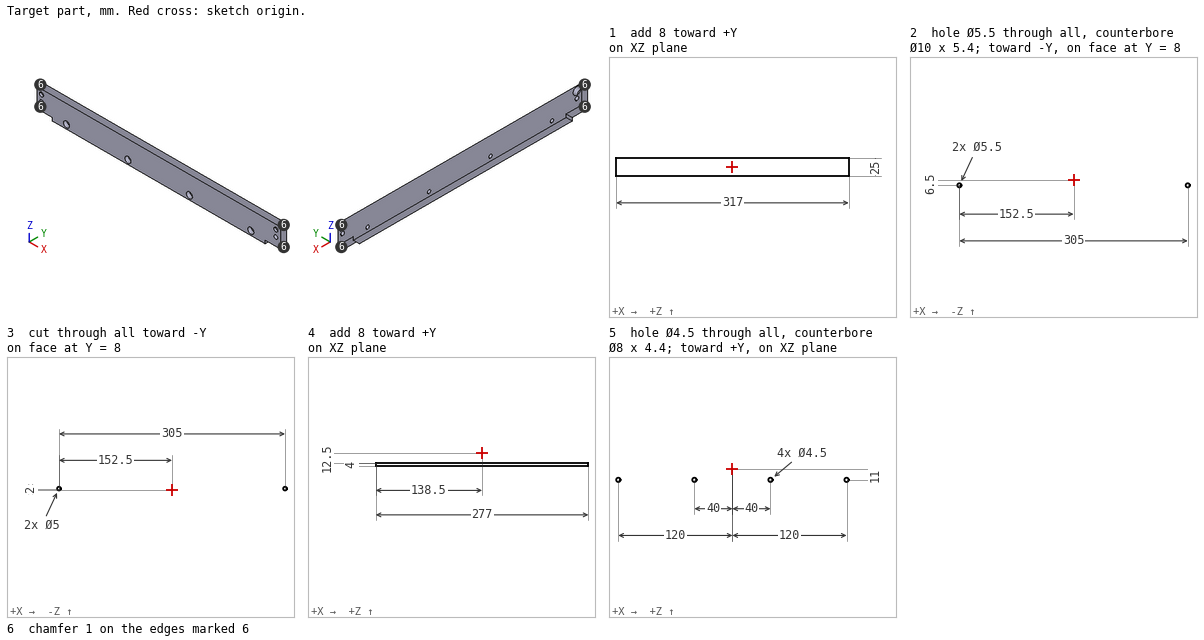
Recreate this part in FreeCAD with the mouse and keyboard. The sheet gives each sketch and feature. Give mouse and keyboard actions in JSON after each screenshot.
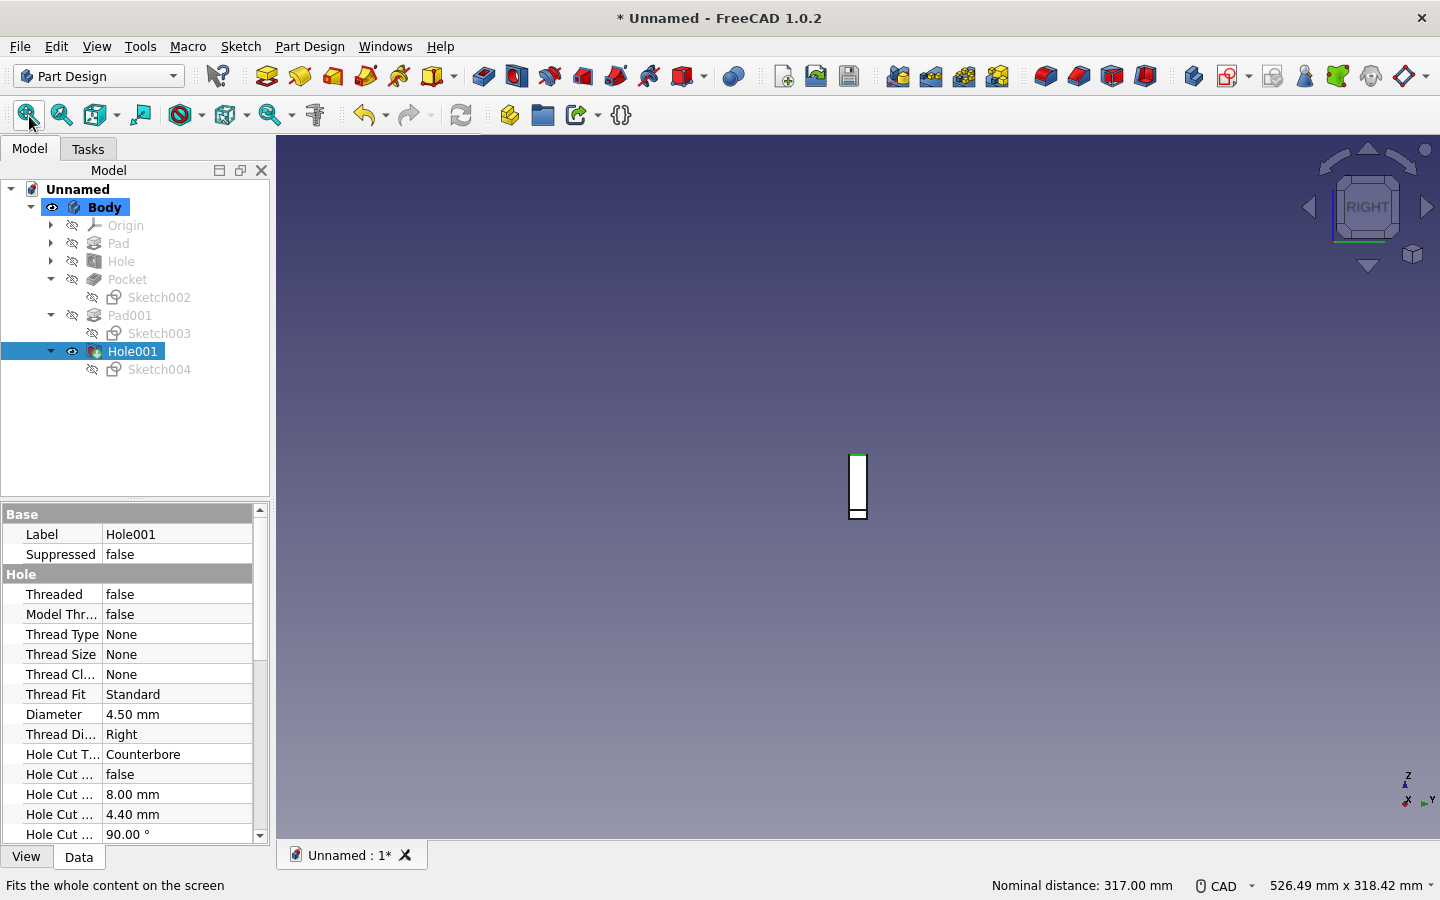
{"action": "left_click", "coordinate": [858, 509], "text": "ctrl"}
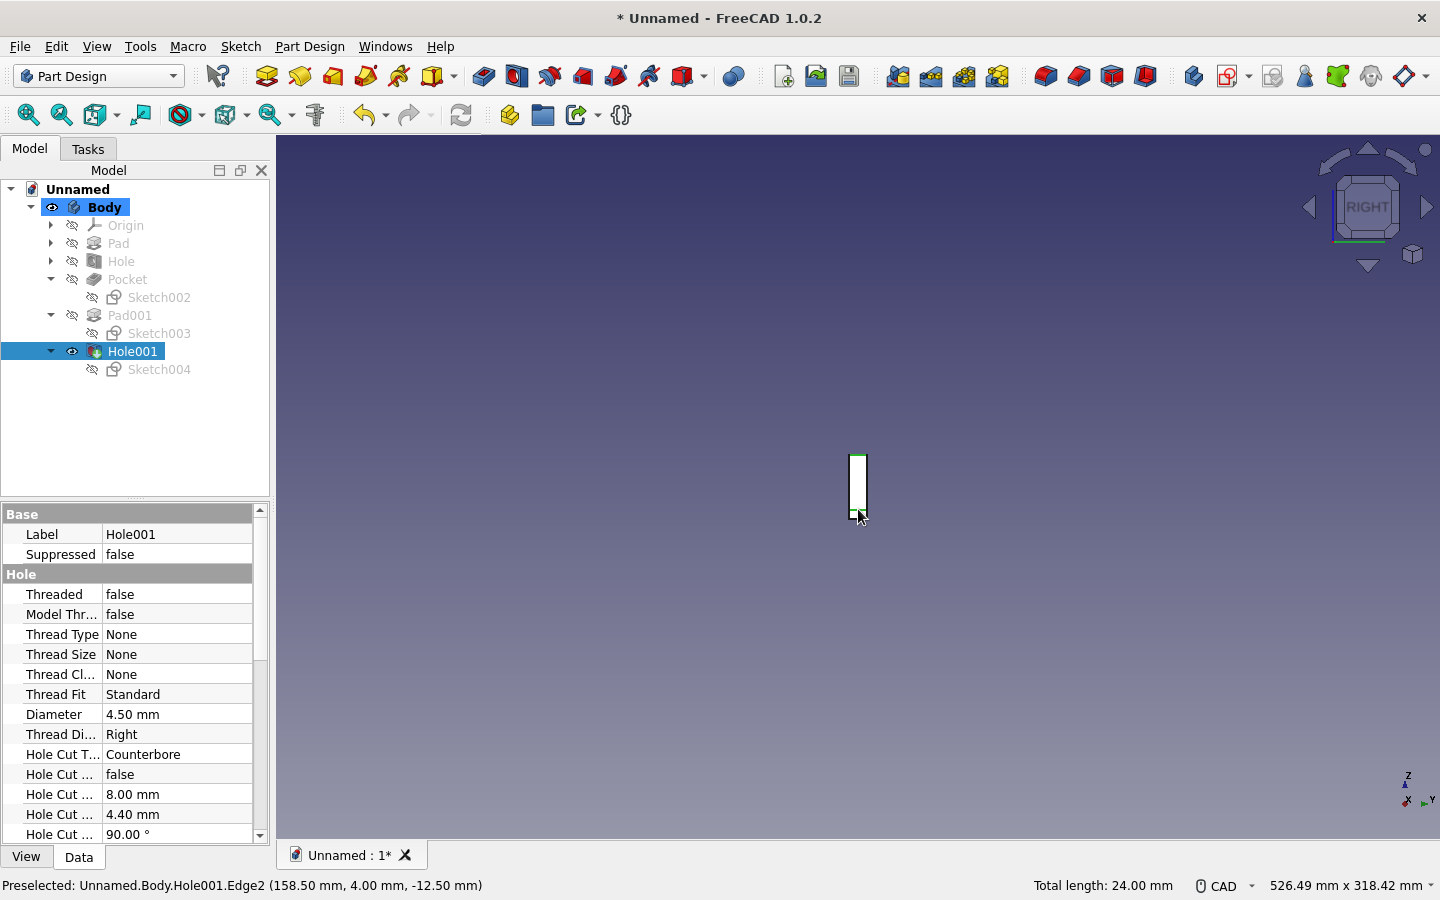
{"action": "scroll", "coordinate": [858, 509], "scroll_direction": "up", "scroll_amount": 5}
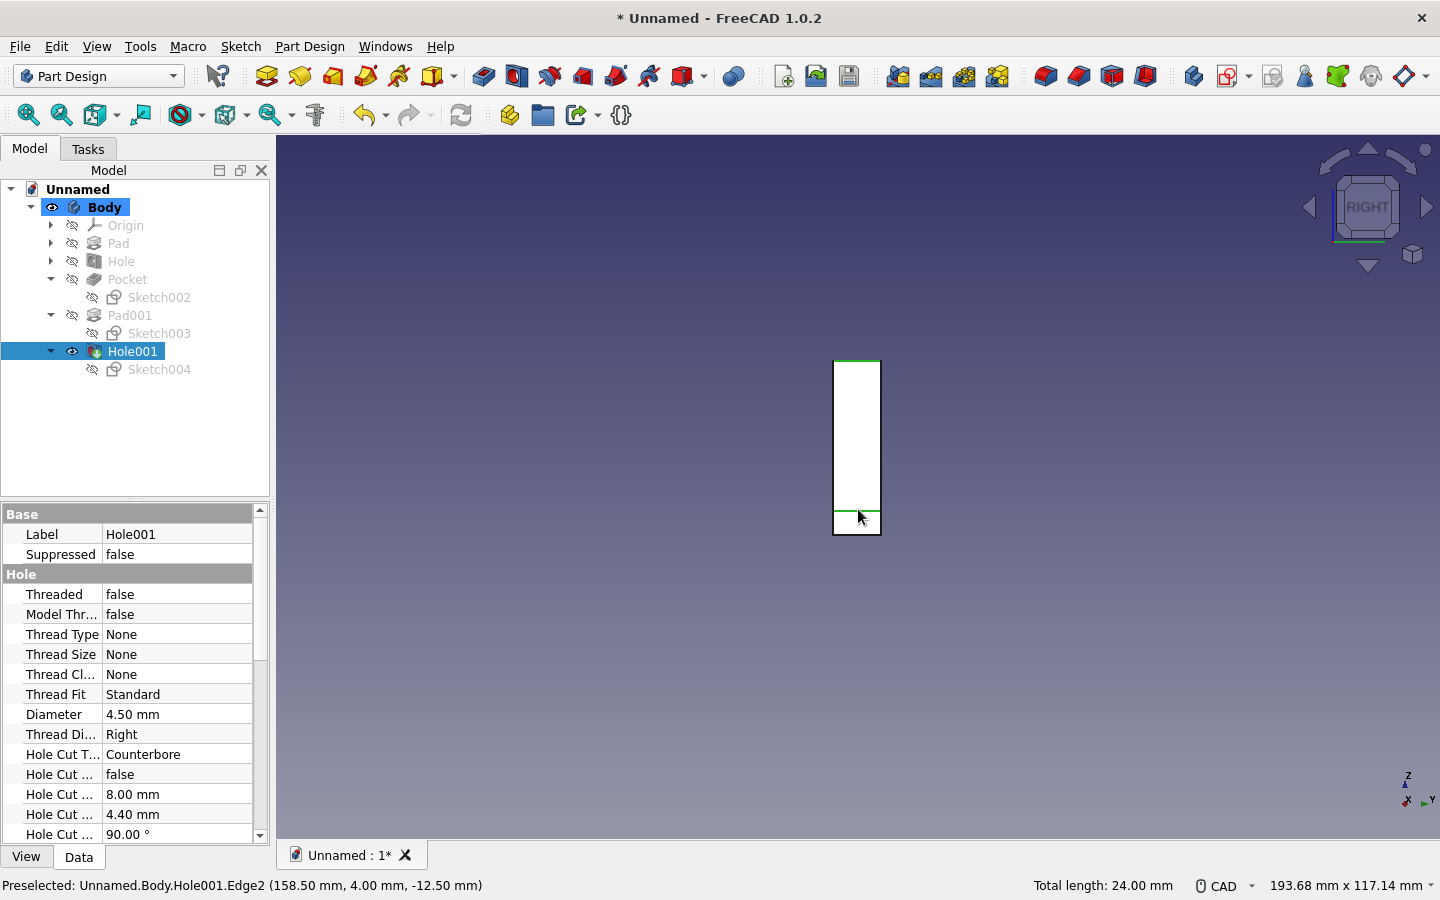
{"action": "left_click", "coordinate": [29, 116]}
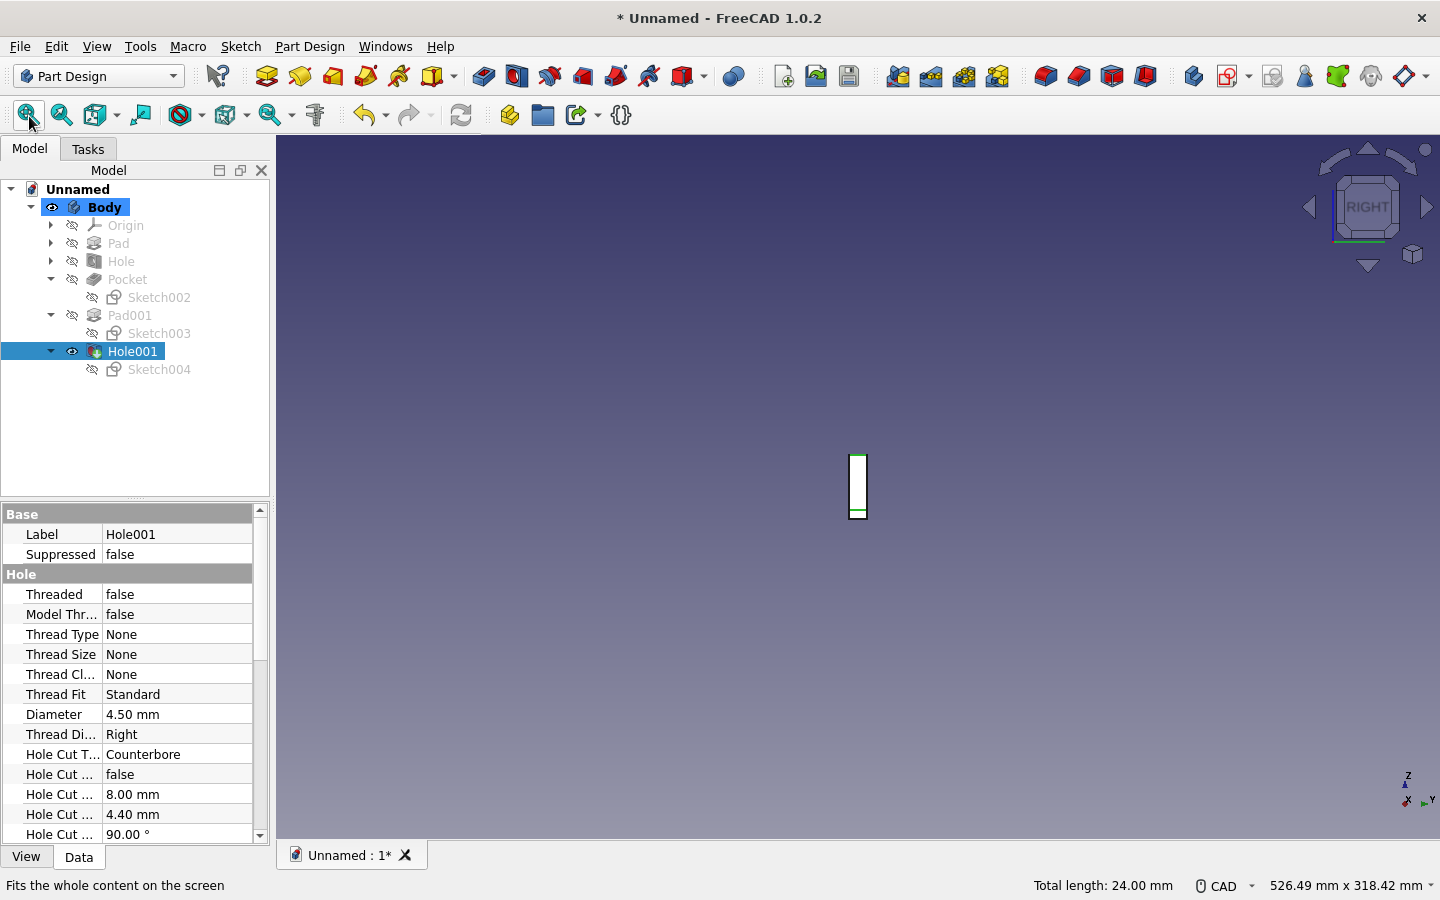
{"action": "key", "text": "5"}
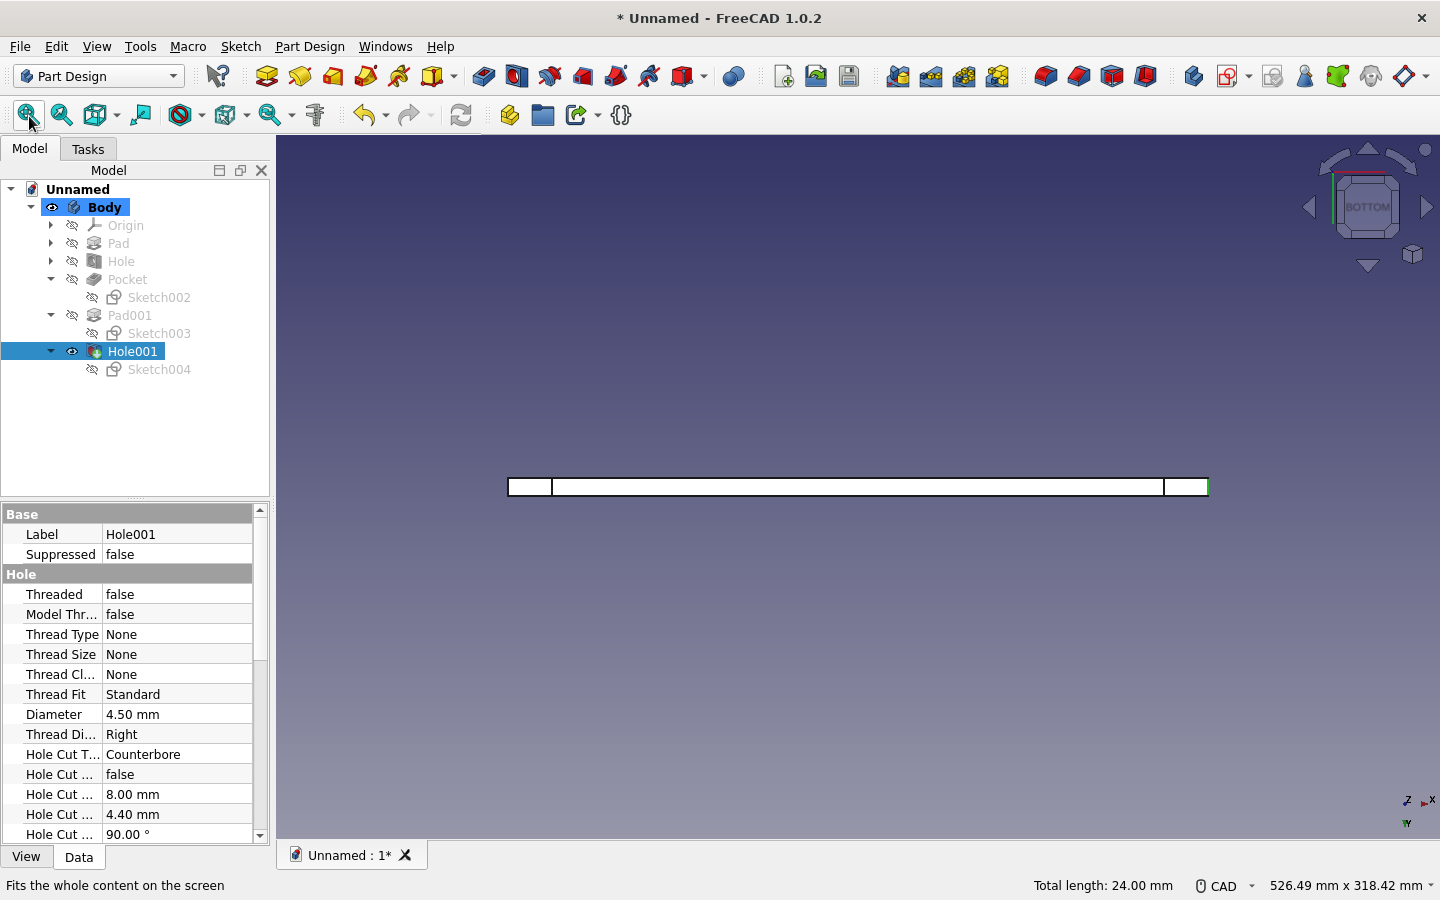
{"action": "left_click", "coordinate": [508, 486], "text": "ctrl"}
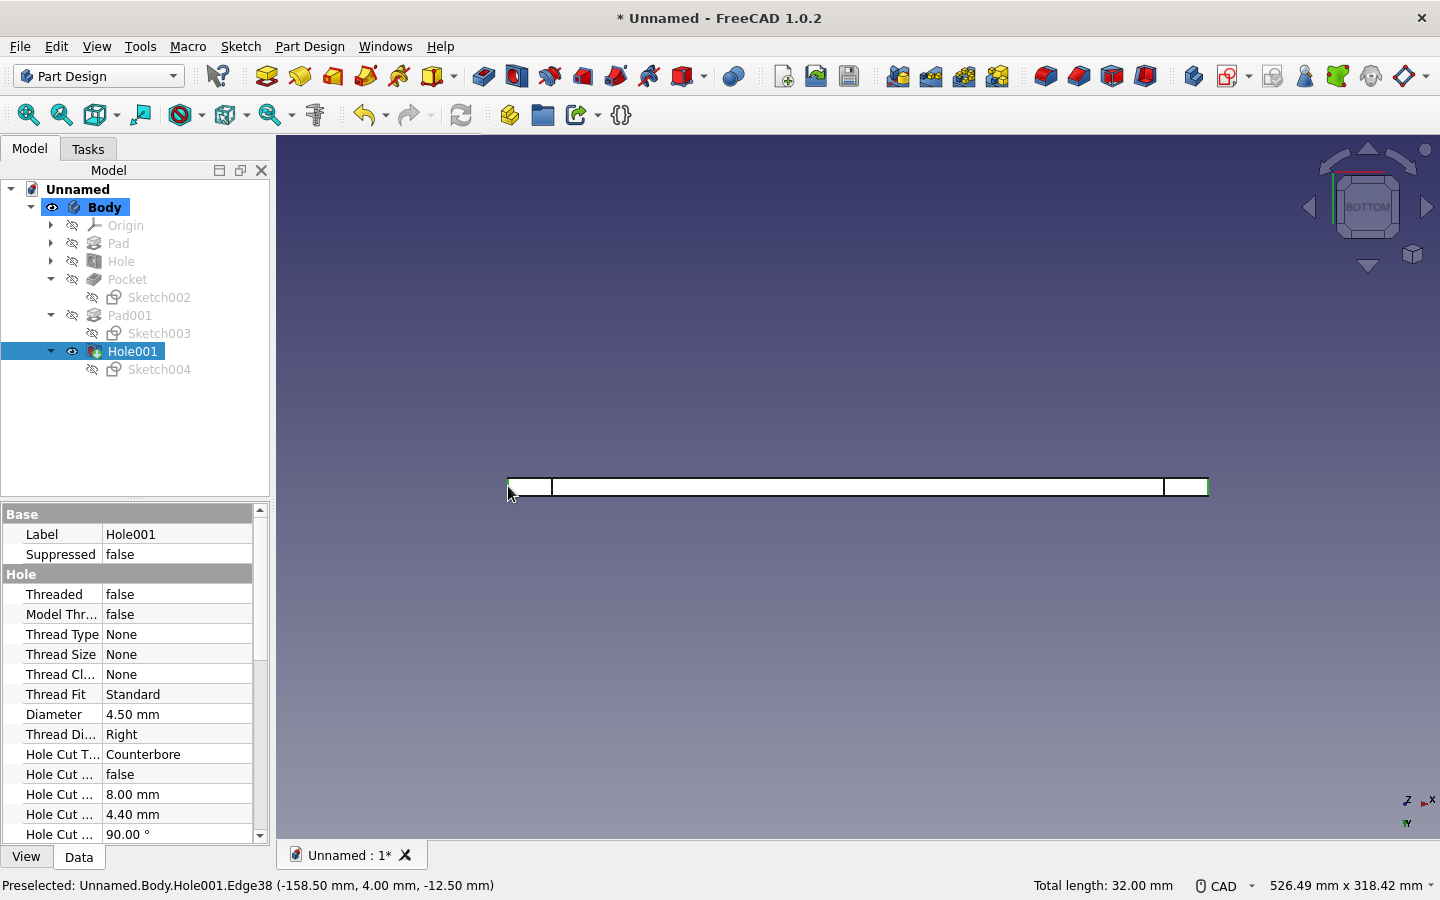
{"action": "left_click", "coordinate": [1079, 76]}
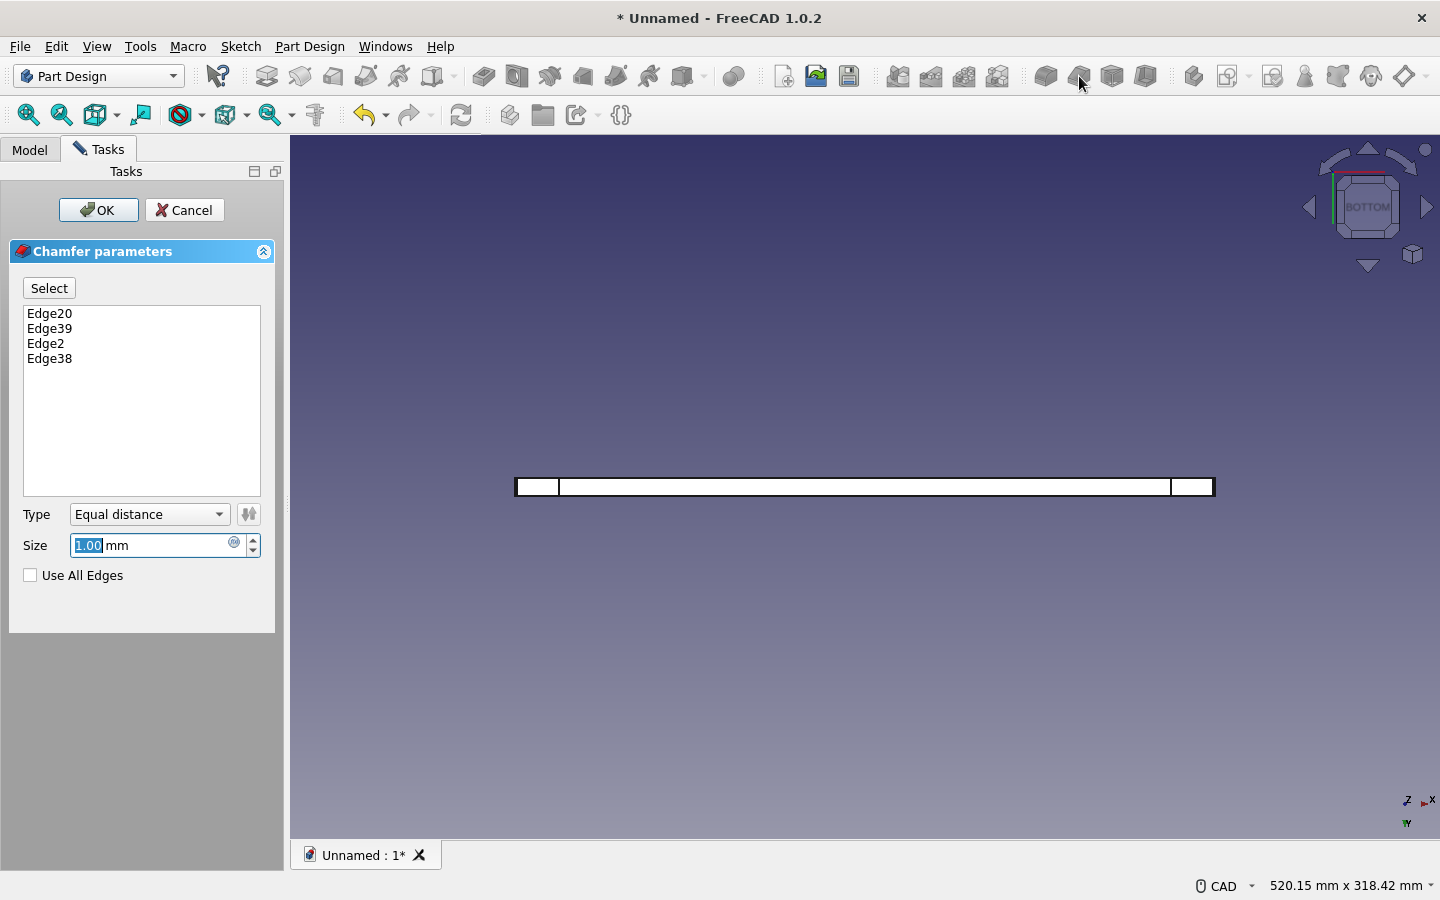
{"action": "type", "text": "1"}
{"action": "key", "text": "Tab"}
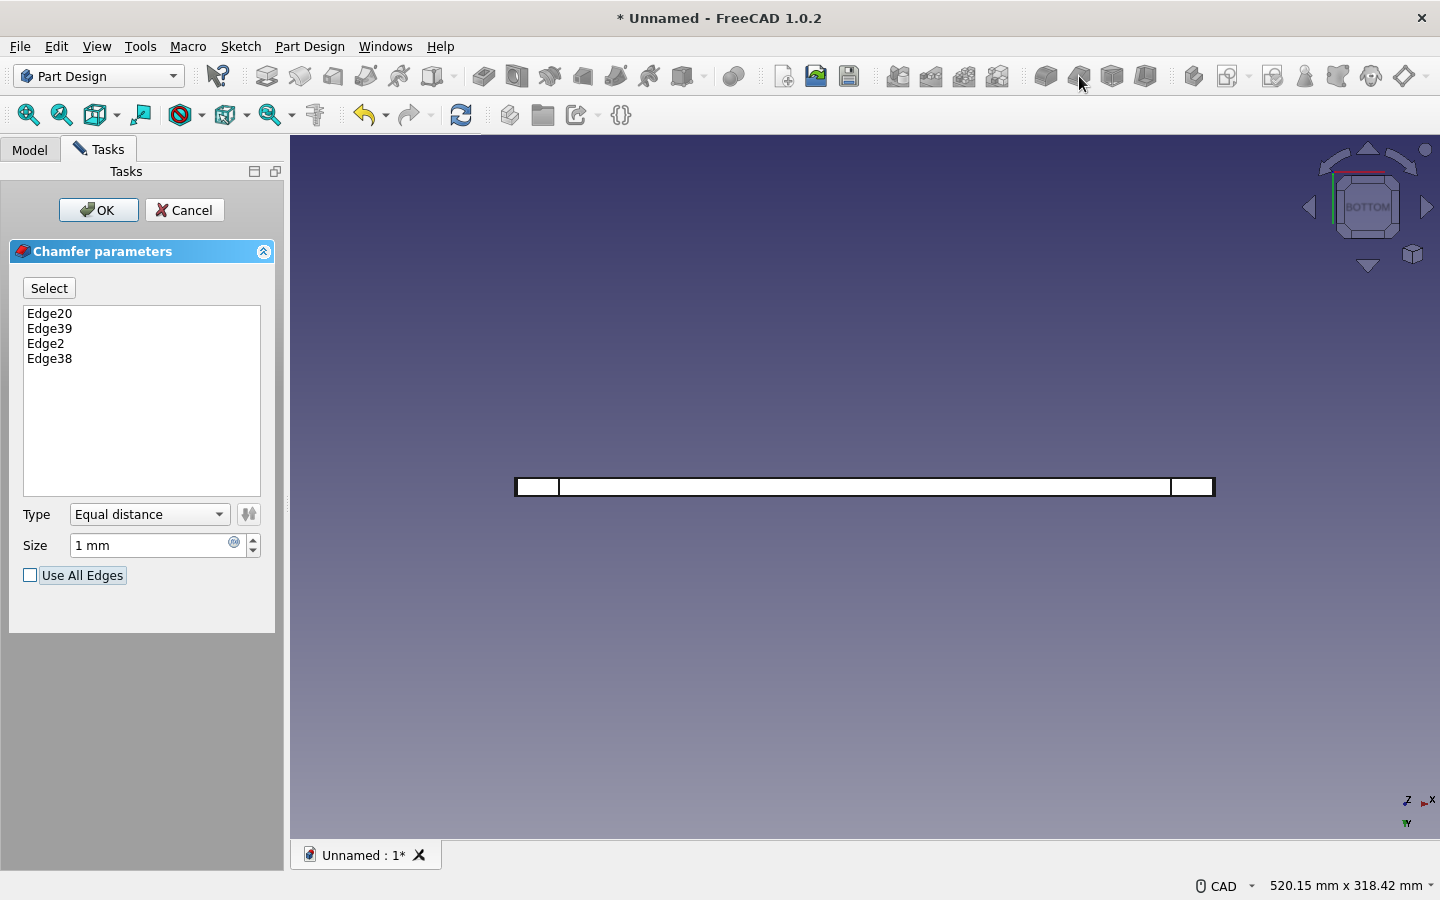
{"action": "left_click", "coordinate": [99, 210]}